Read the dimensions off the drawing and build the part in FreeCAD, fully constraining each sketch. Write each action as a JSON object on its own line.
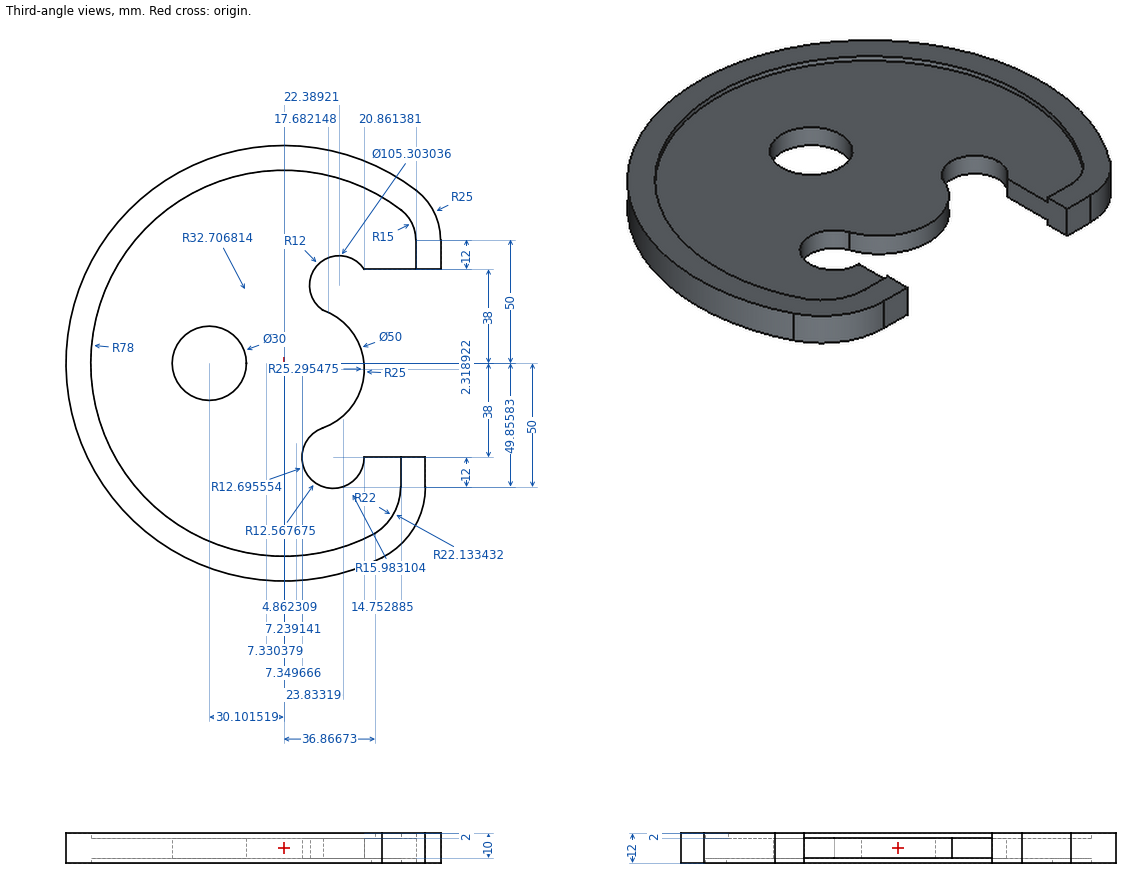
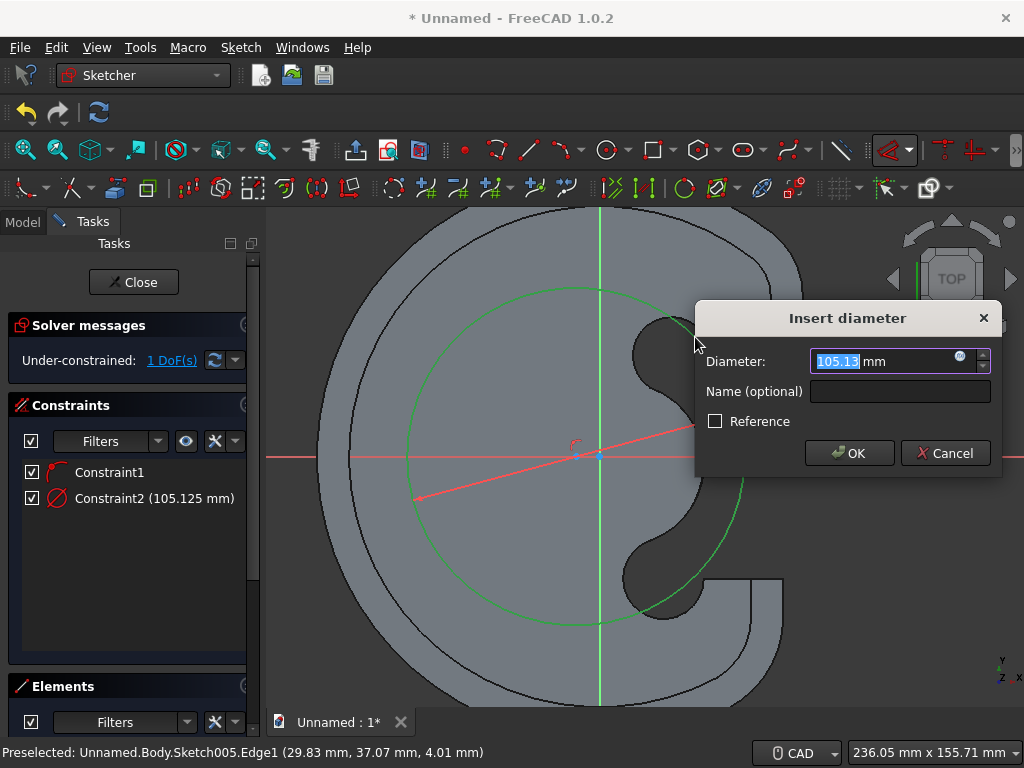
{"action": "type", "text": "105.303036"}
{"action": "key", "text": "Return"}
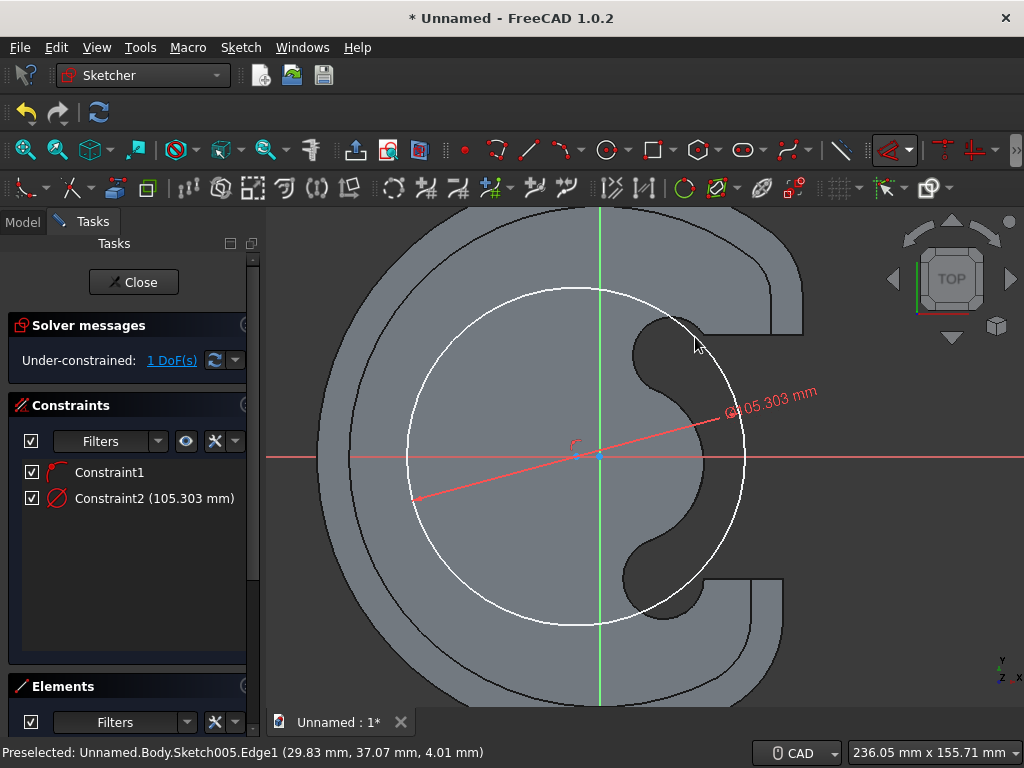
{"action": "scroll", "coordinate": [576, 457], "scroll_direction": "up", "scroll_amount": 3}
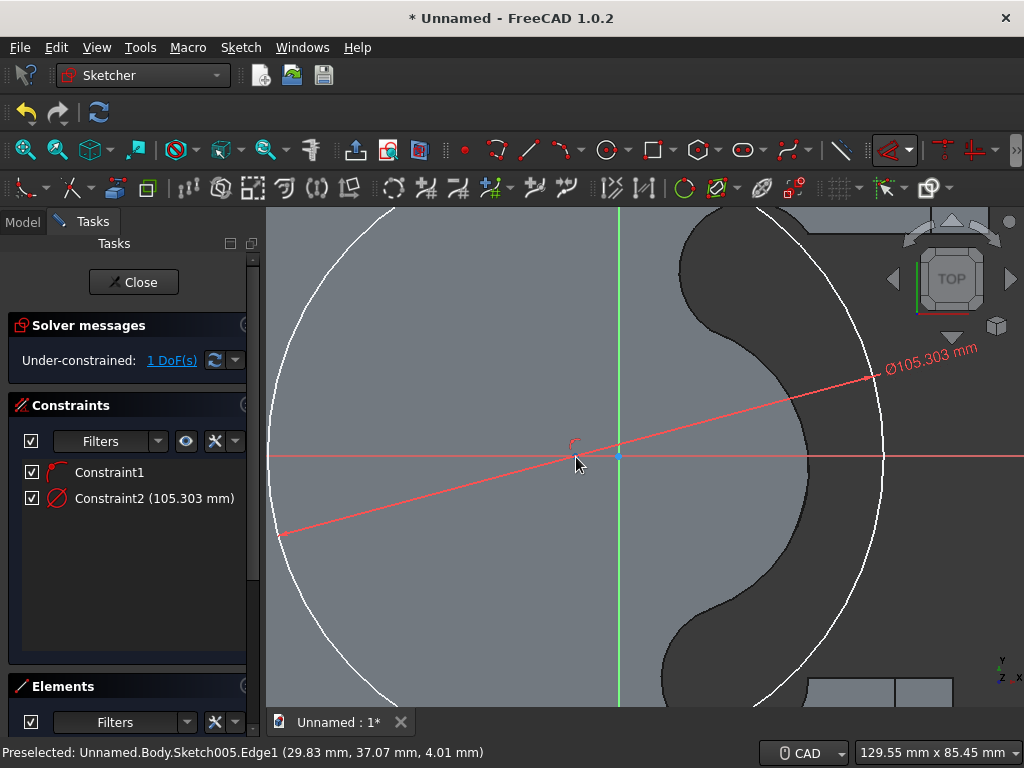
{"action": "left_click", "coordinate": [576, 456]}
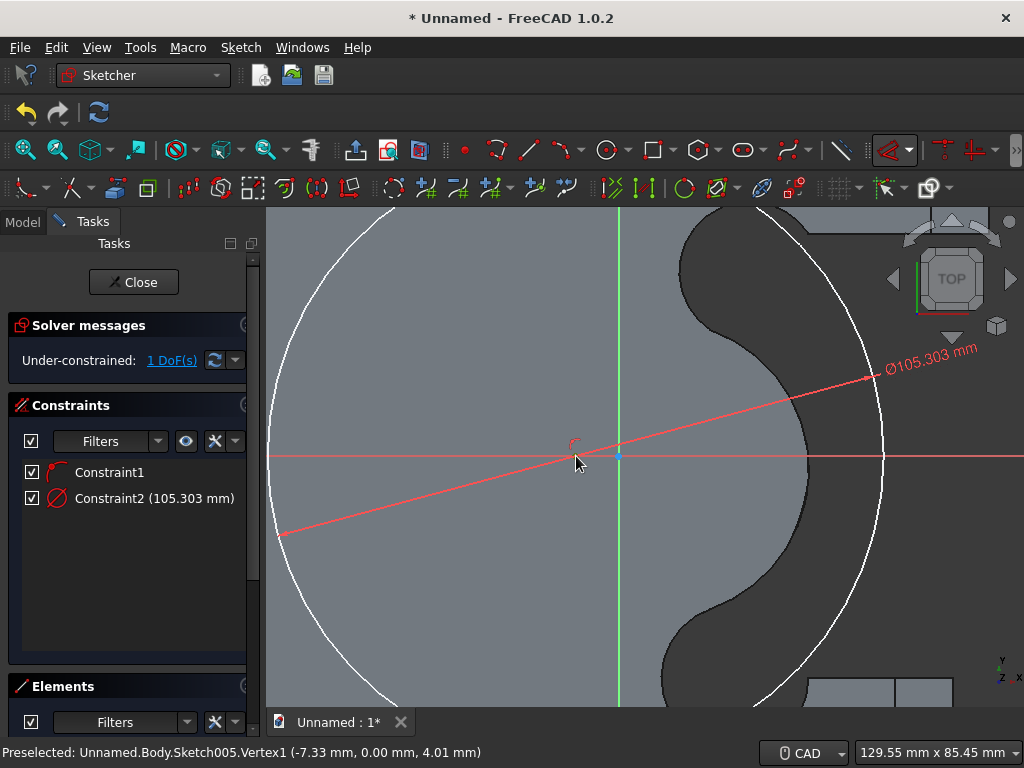
{"action": "key", "text": "l"}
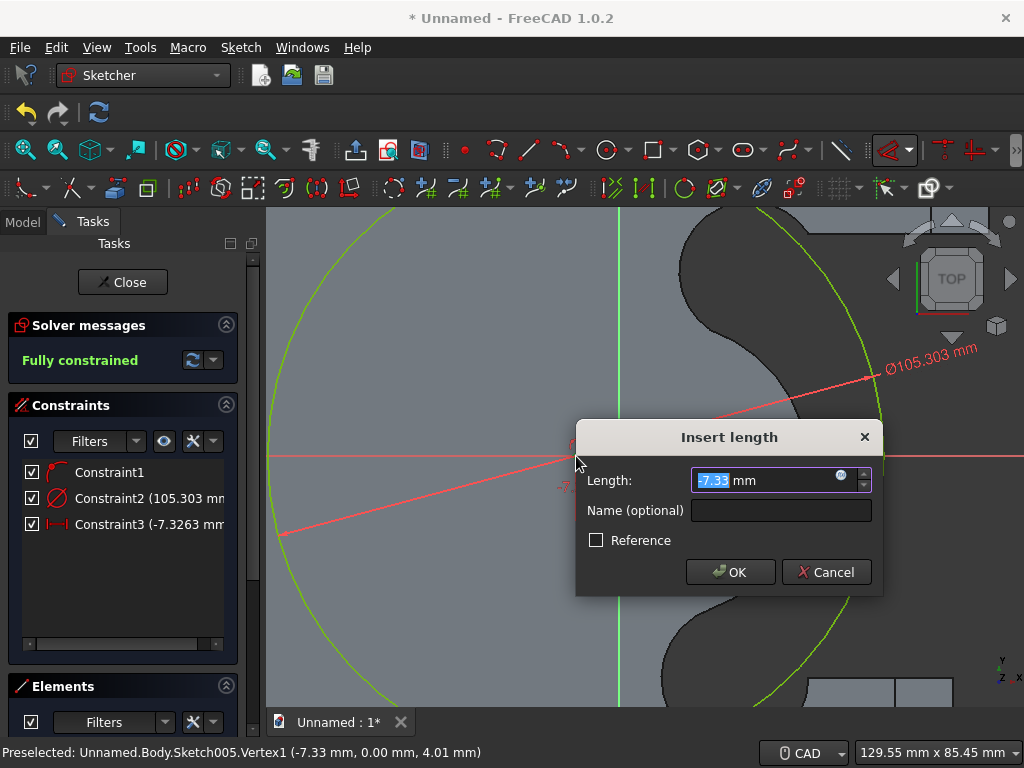
{"action": "type", "text": "-7.330379"}
{"action": "key", "text": "Return"}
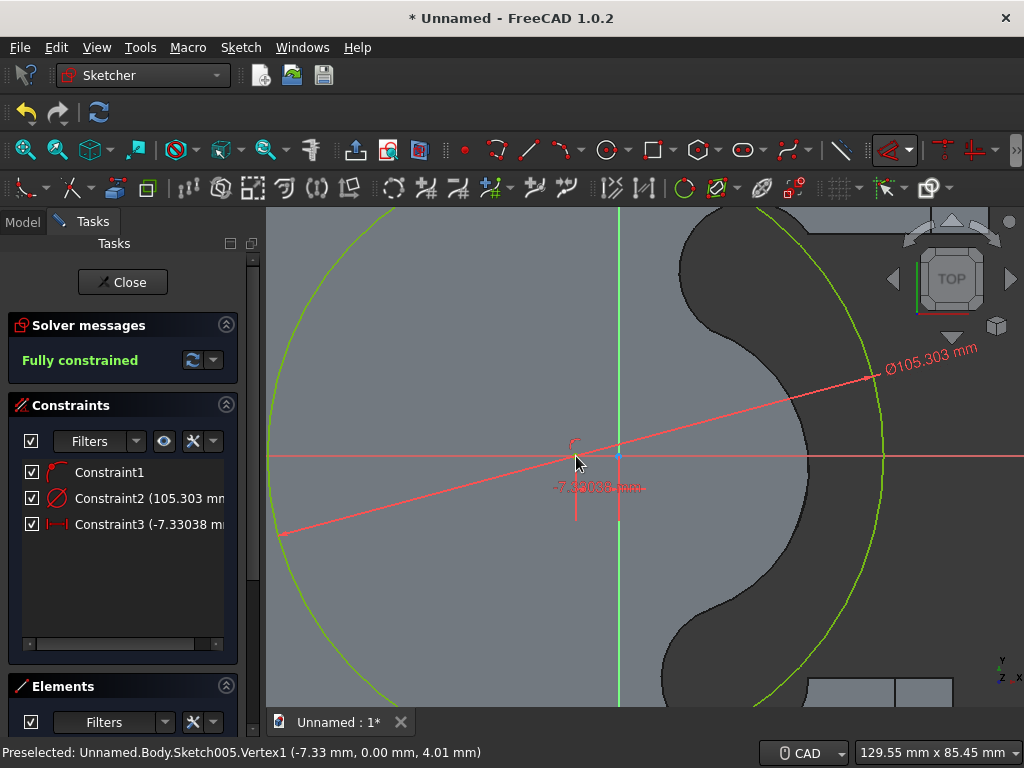
{"action": "left_click", "coordinate": [123, 282]}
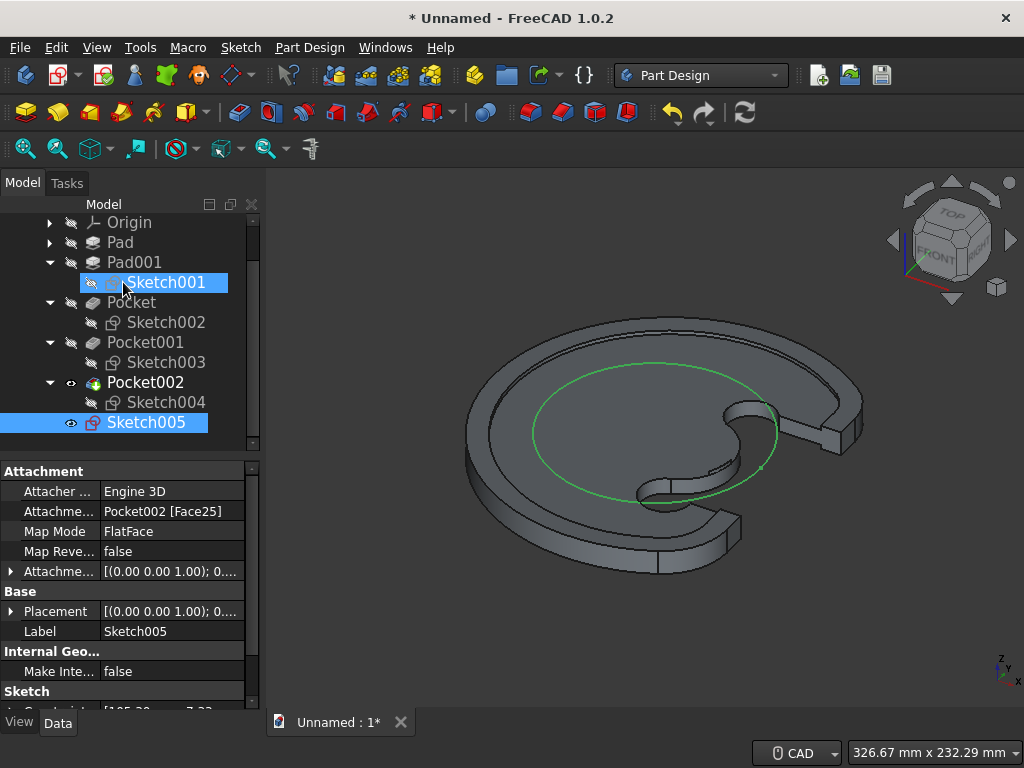
{"action": "left_click", "coordinate": [240, 112]}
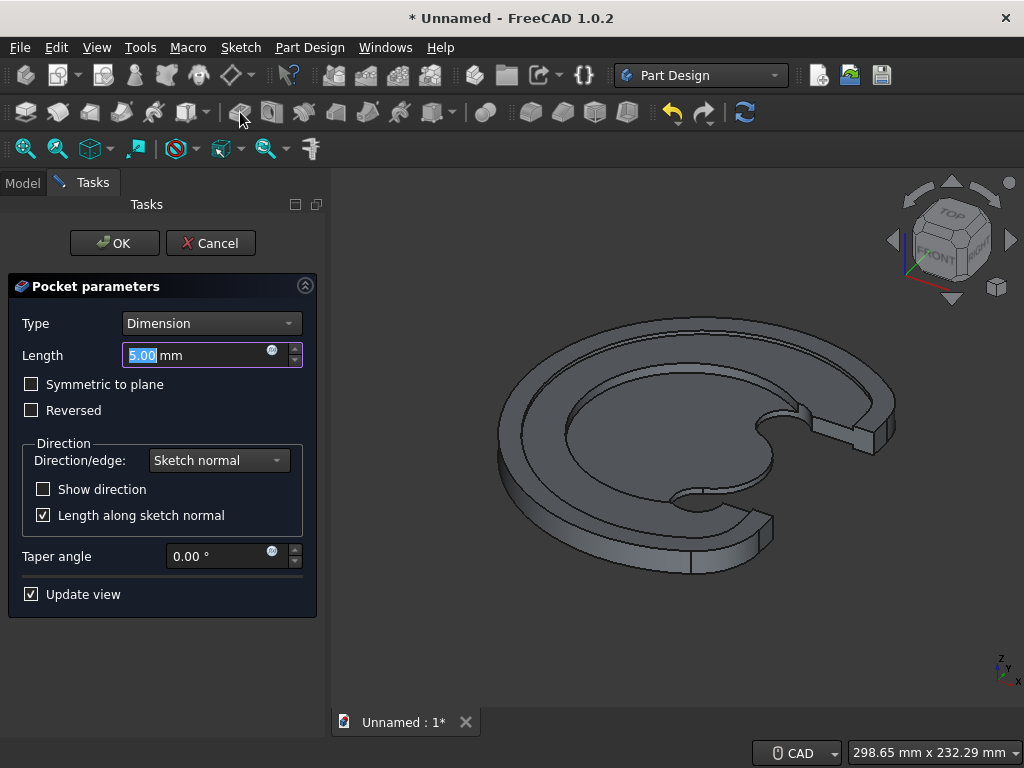
{"action": "type", "text": "2"}
{"action": "key", "text": "Tab"}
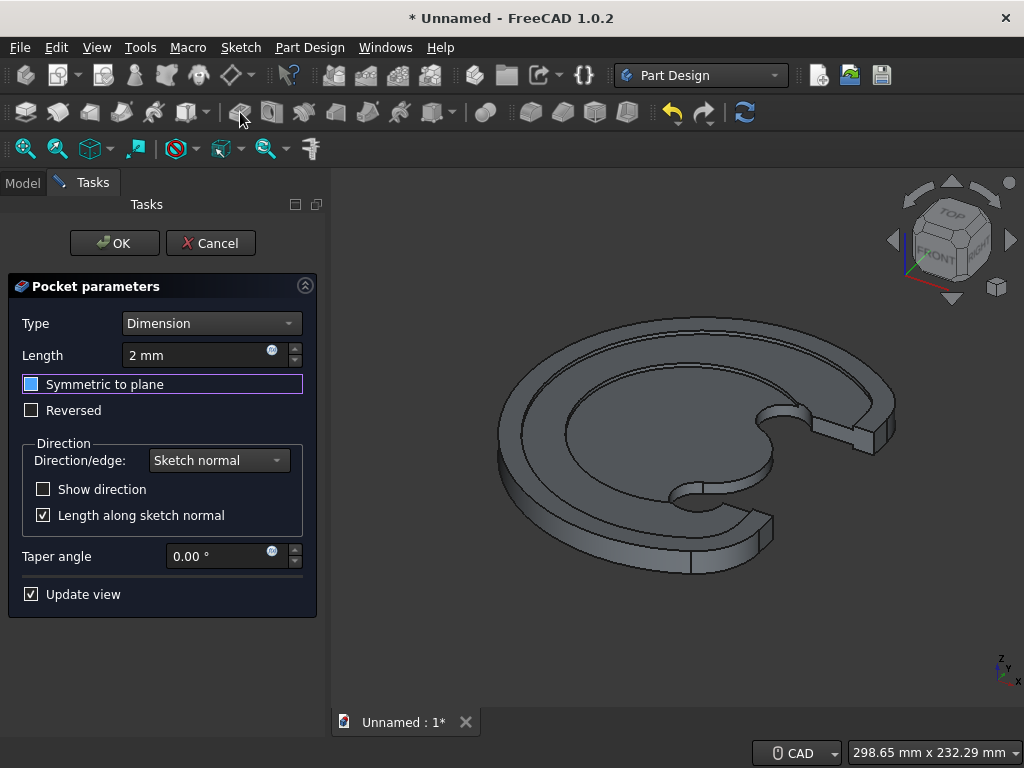
{"action": "left_click", "coordinate": [30, 410]}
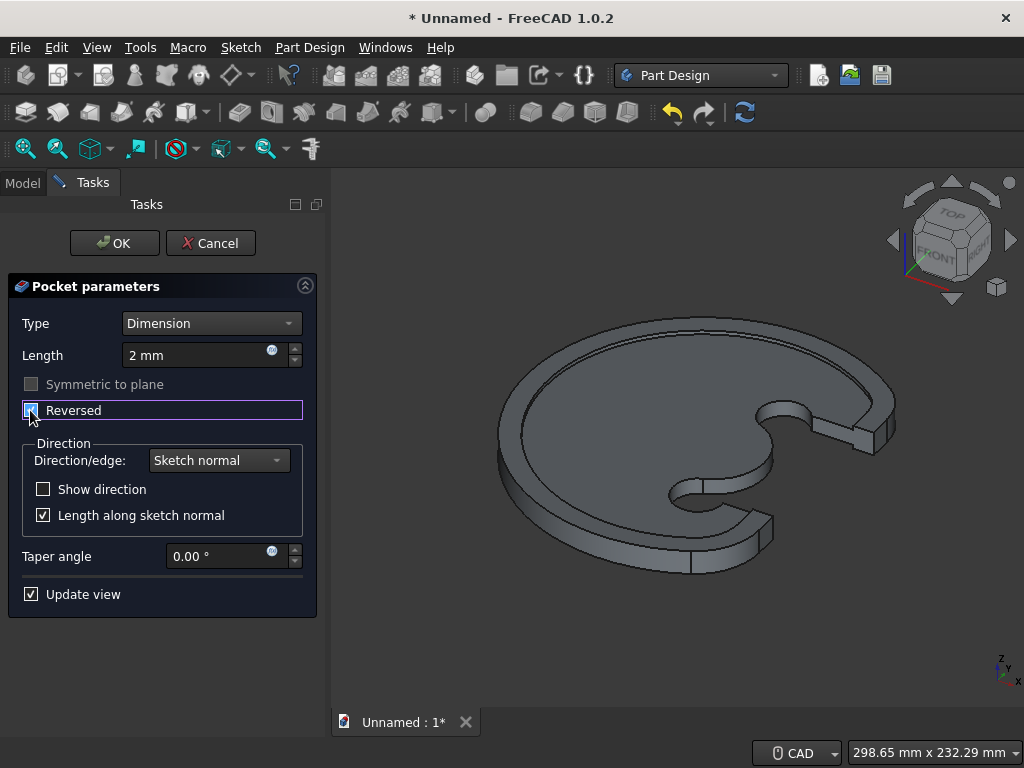
{"action": "left_click", "coordinate": [115, 243]}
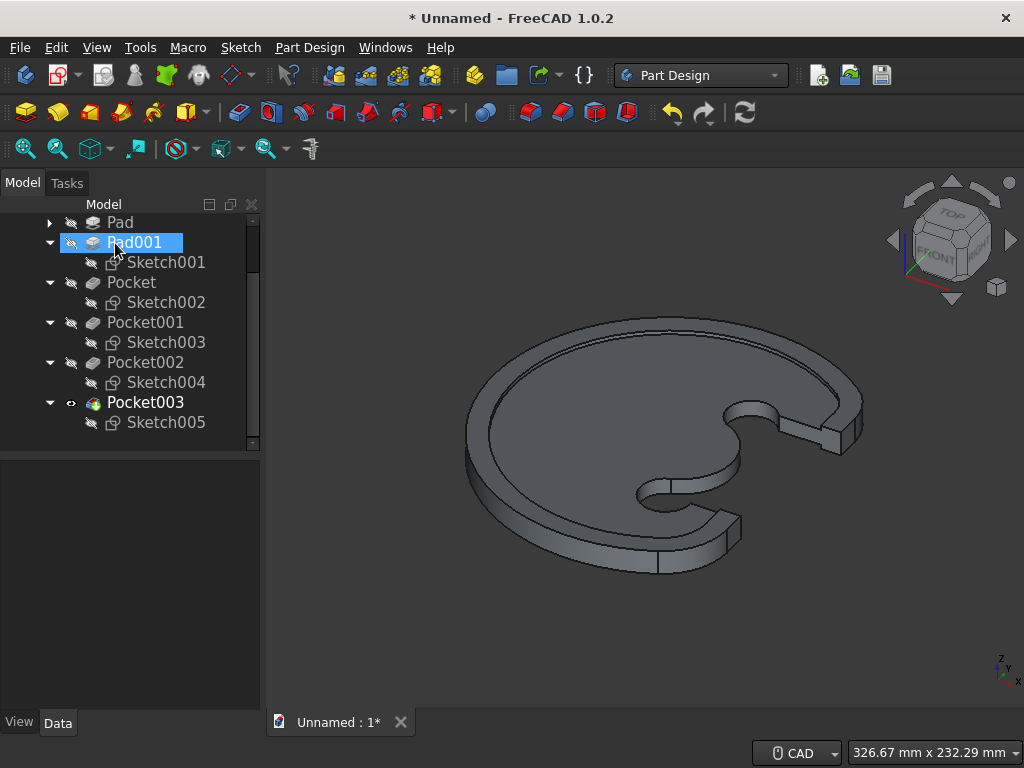
{"action": "left_click", "coordinate": [607, 416]}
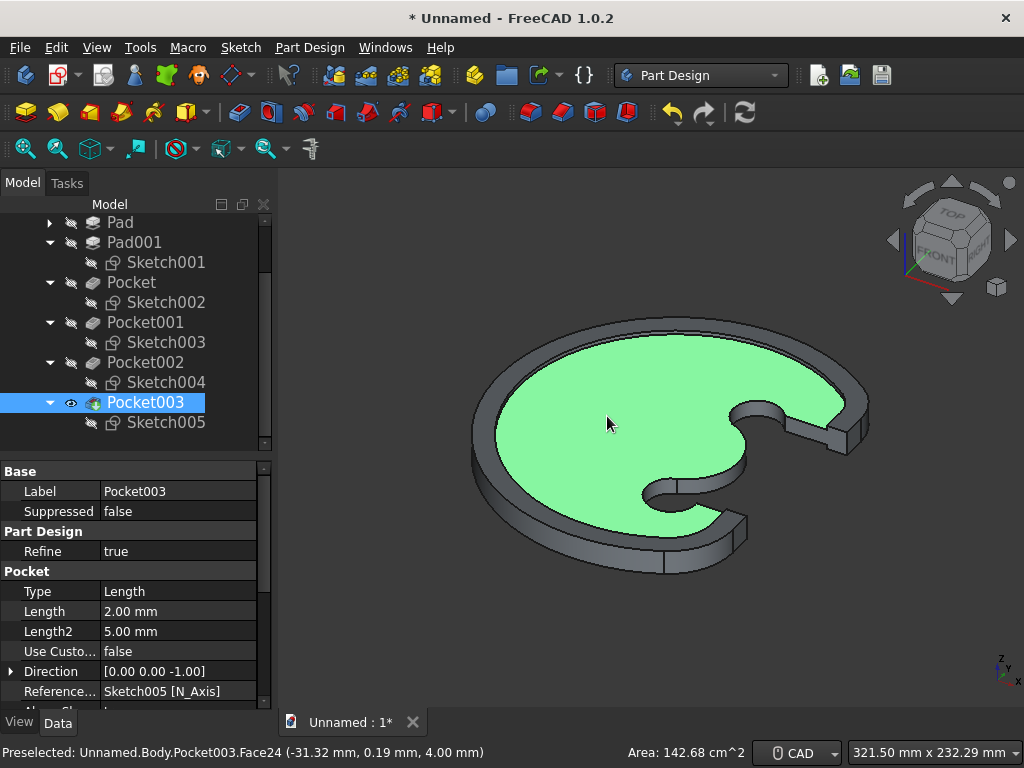
{"action": "left_click", "coordinate": [58, 76]}